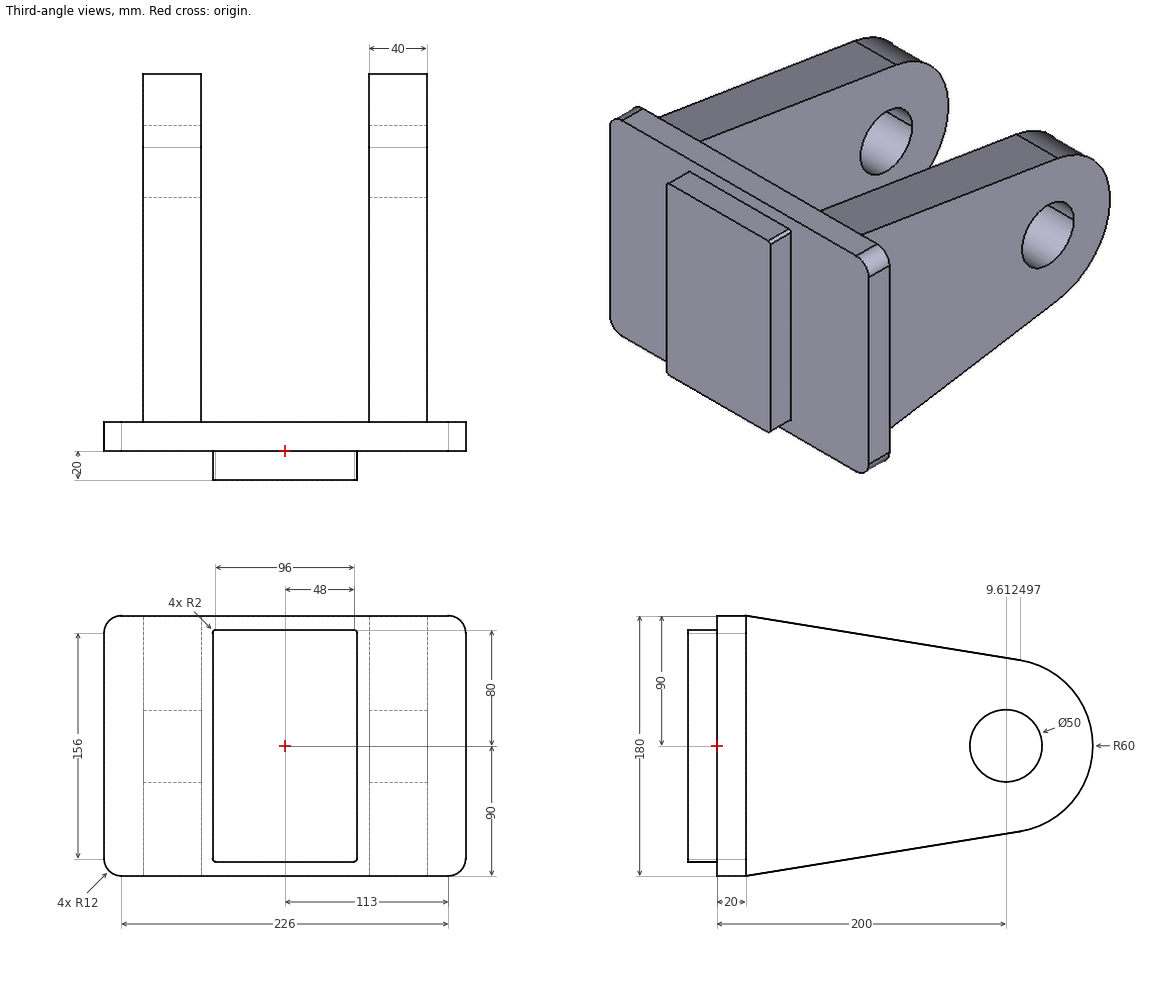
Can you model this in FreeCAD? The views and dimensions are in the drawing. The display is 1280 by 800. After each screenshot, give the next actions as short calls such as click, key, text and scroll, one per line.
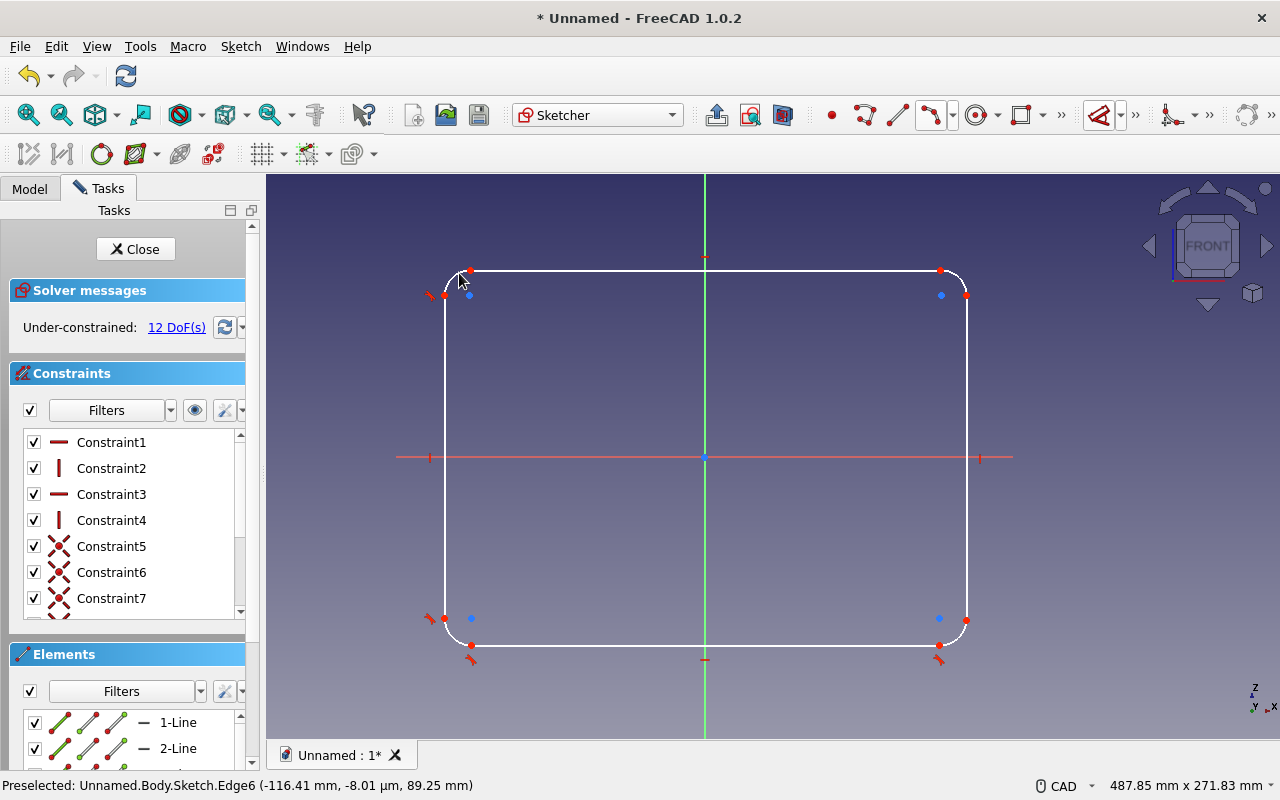
click(611, 271)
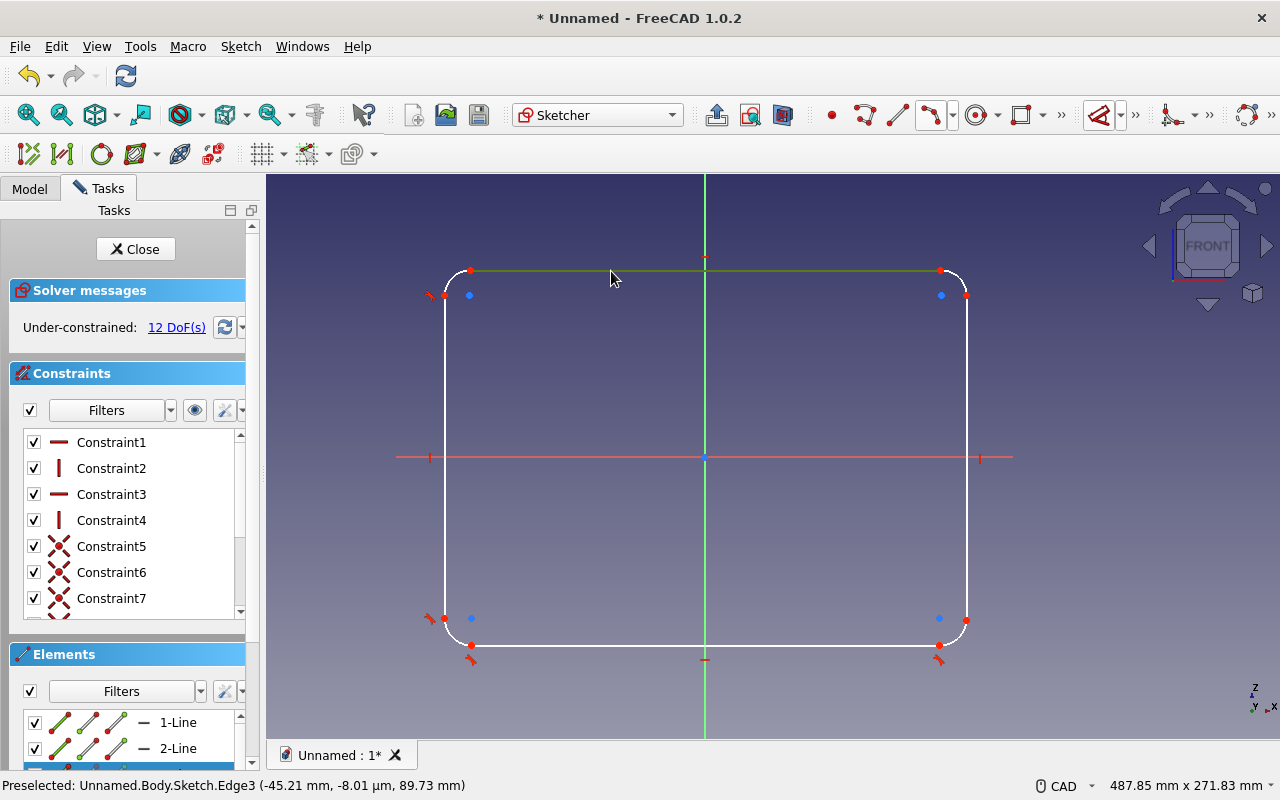
click(459, 273)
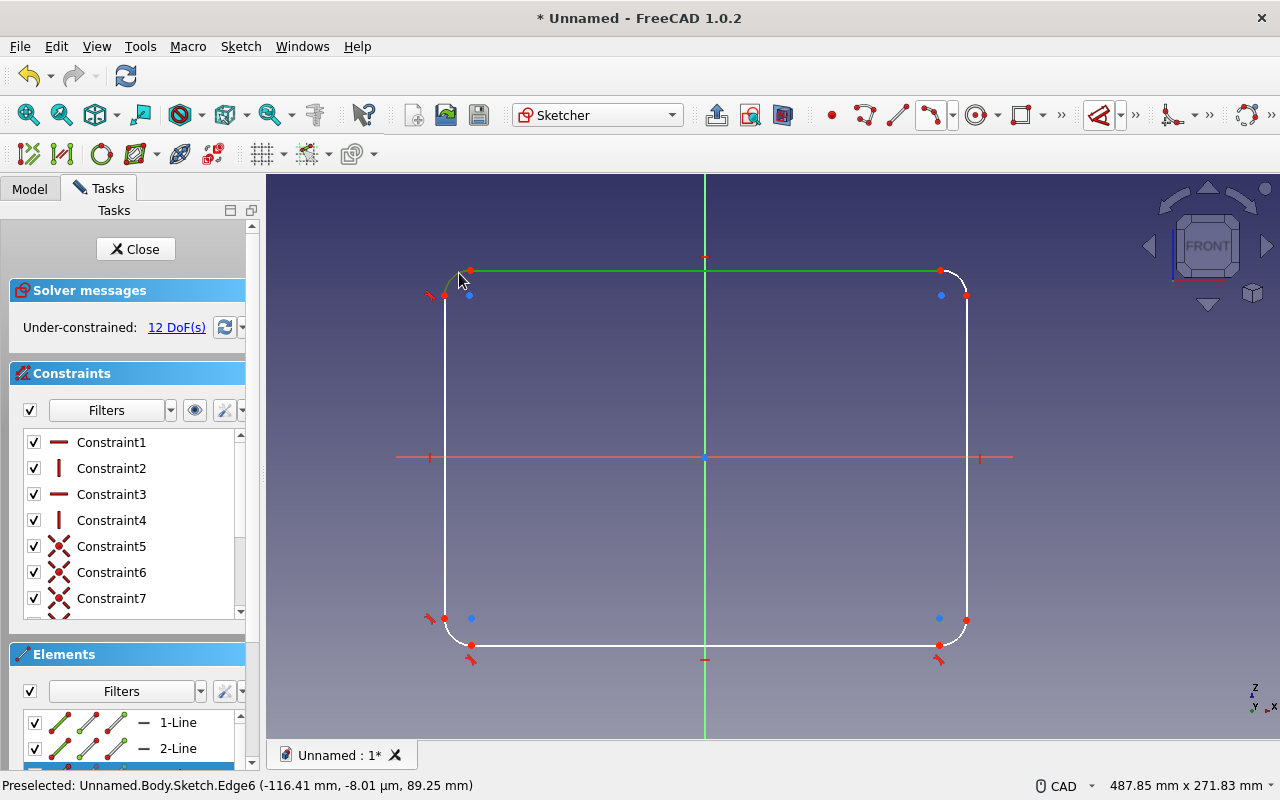
key(t)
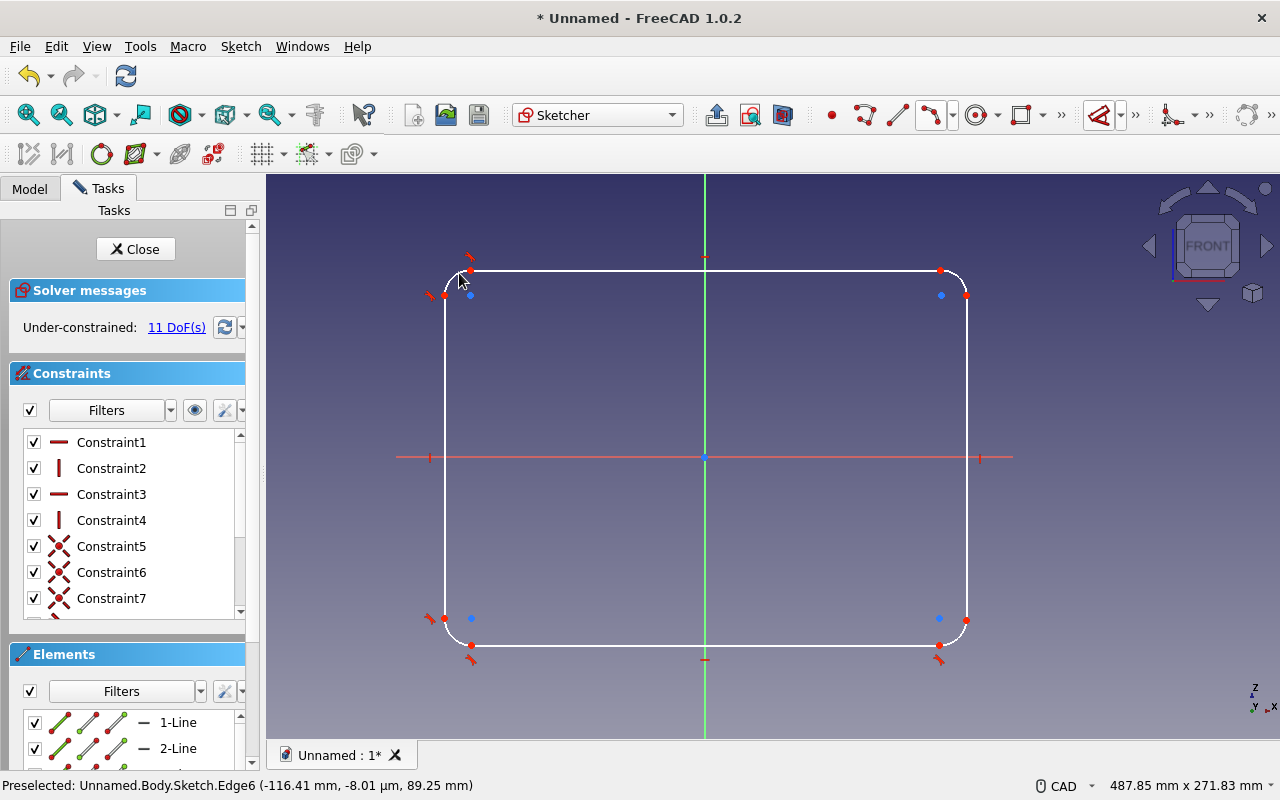
click(611, 271)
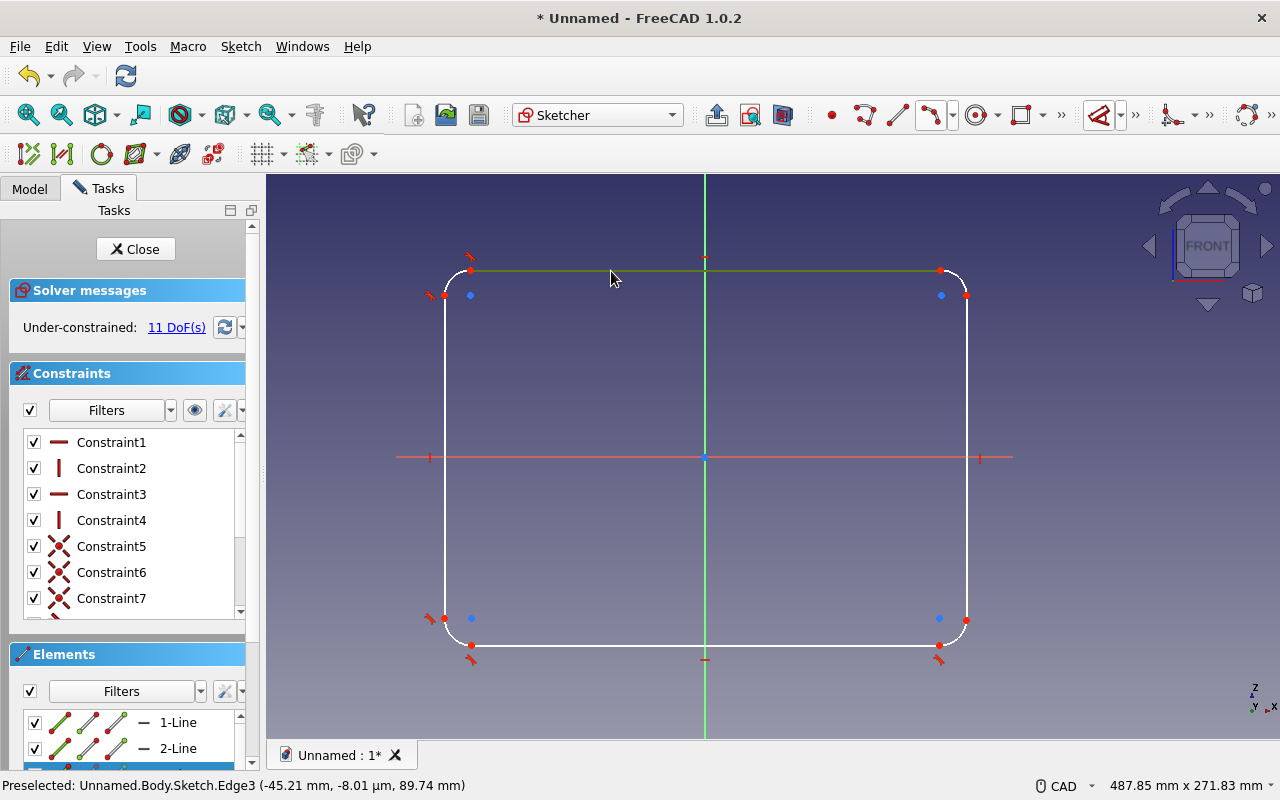
click(964, 284)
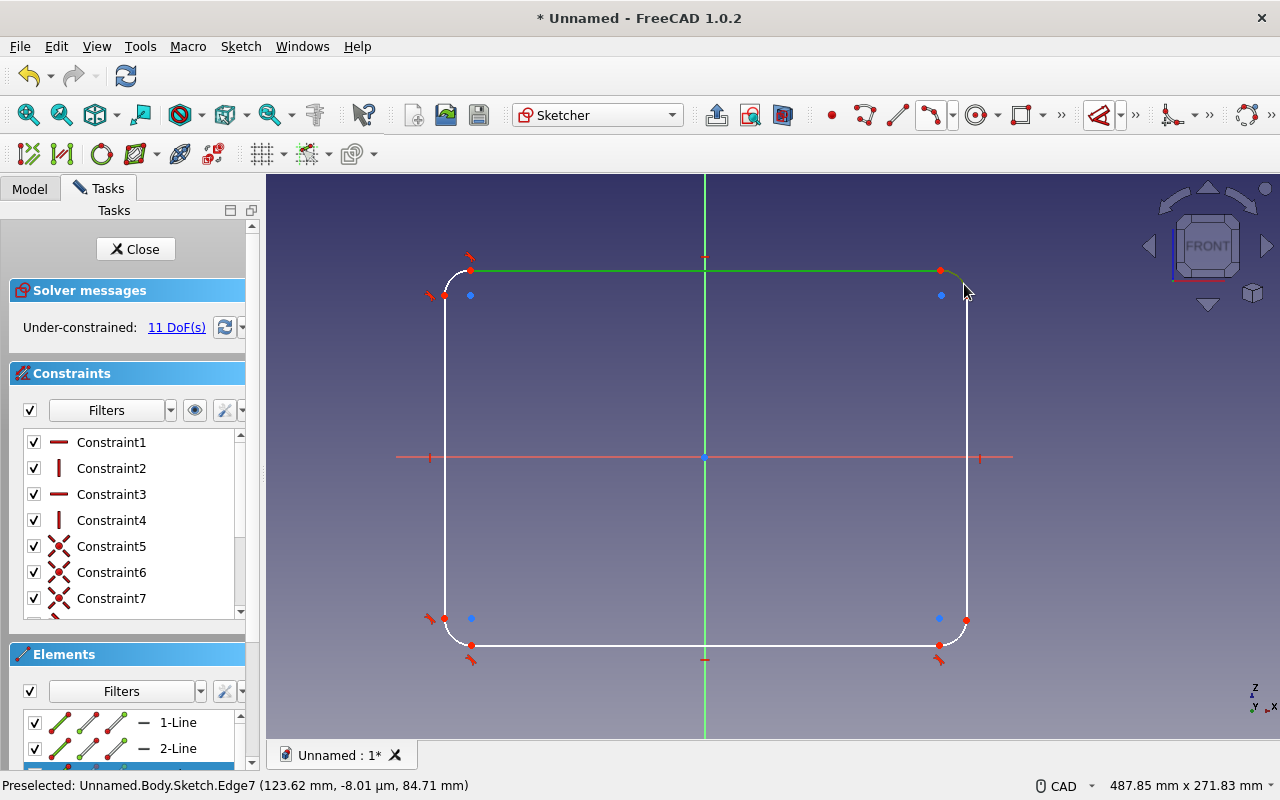
key(t)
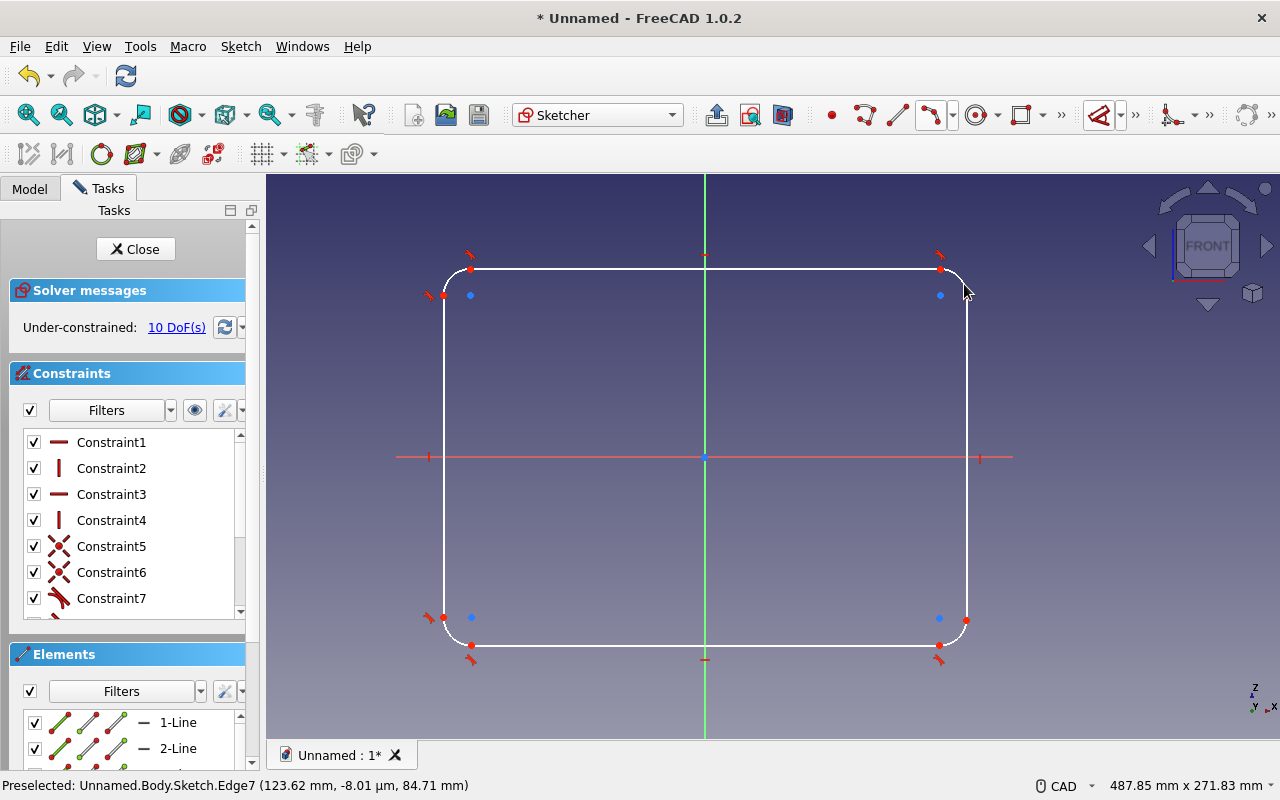
click(967, 393)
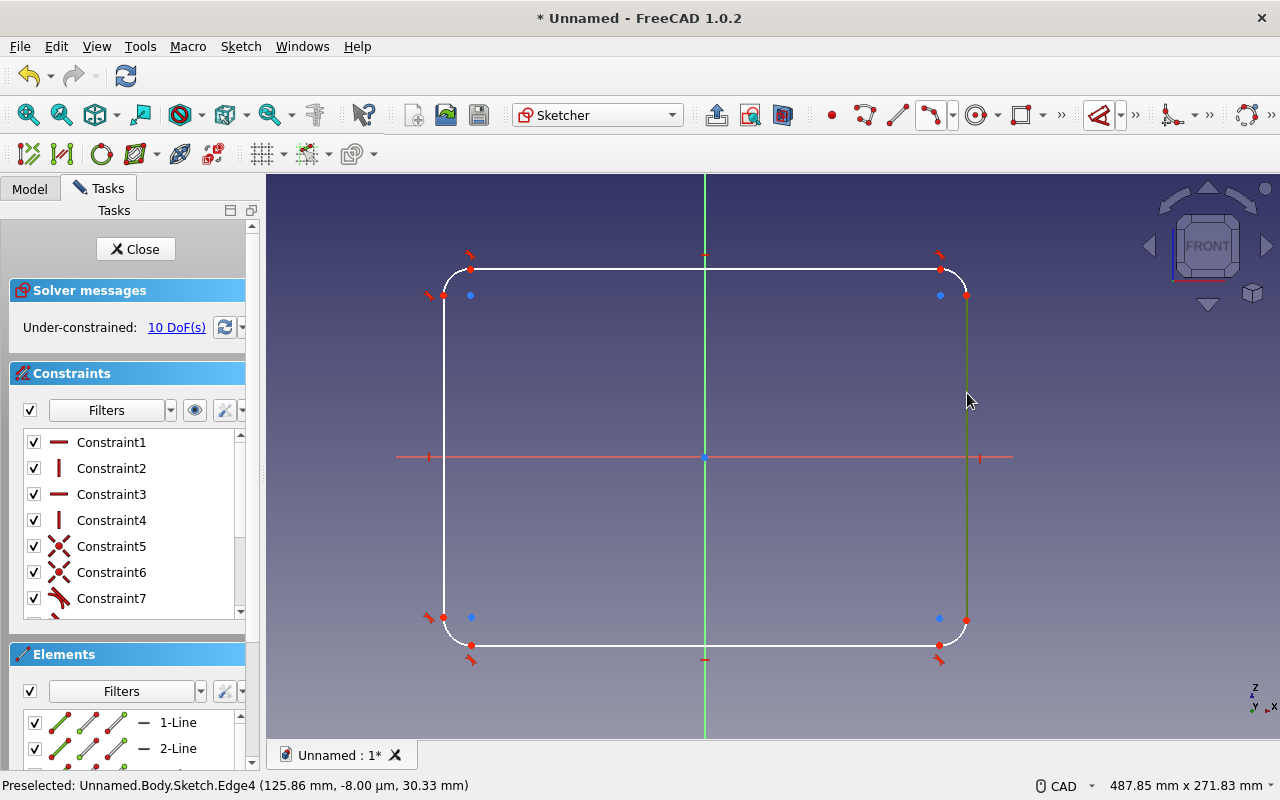
click(964, 284)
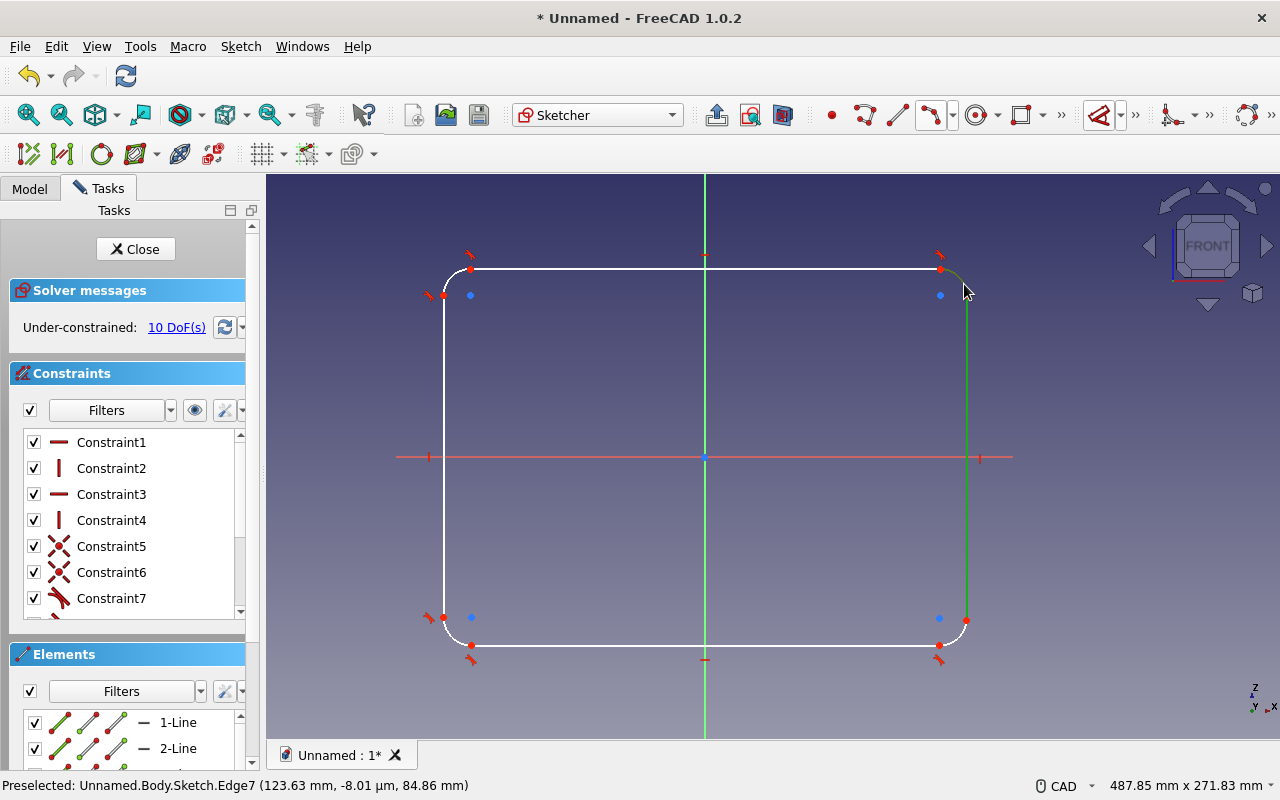
key(t)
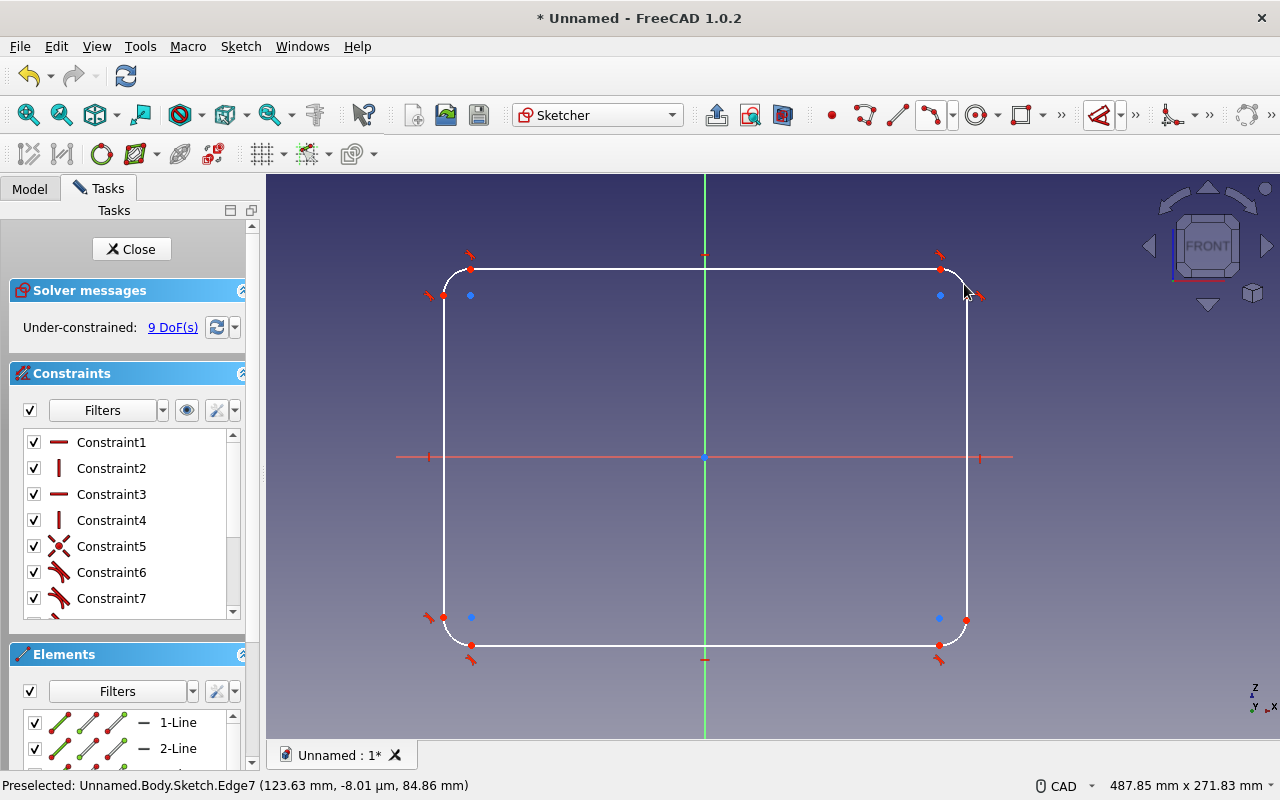
click(967, 393)